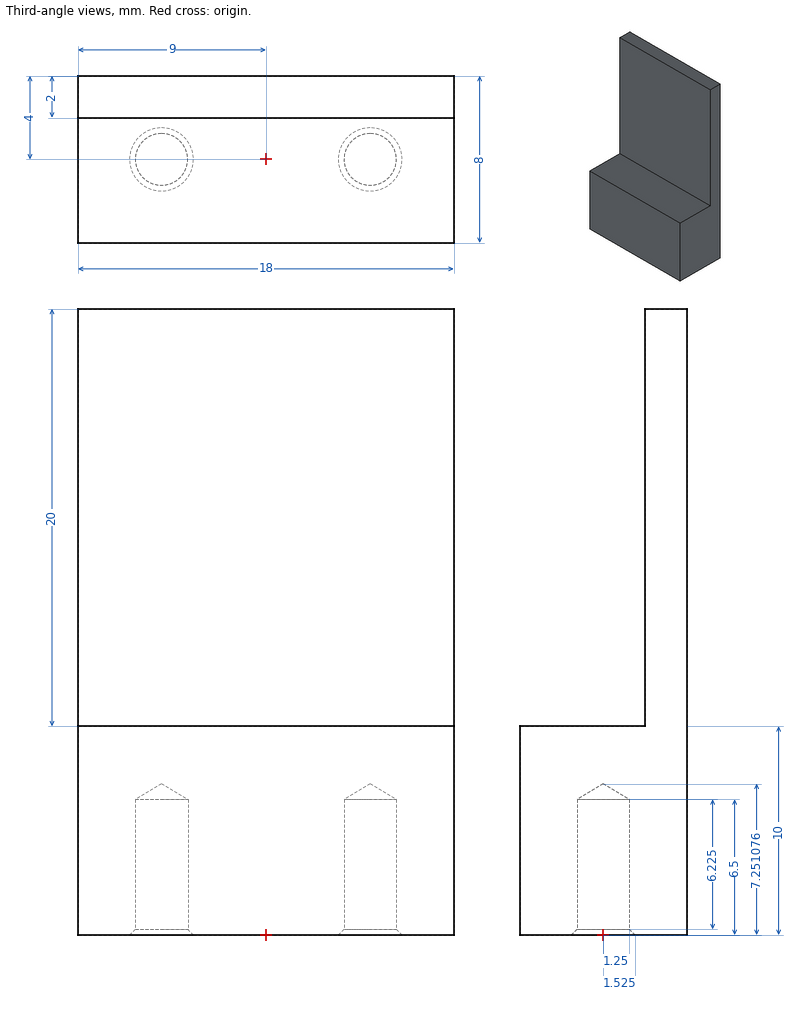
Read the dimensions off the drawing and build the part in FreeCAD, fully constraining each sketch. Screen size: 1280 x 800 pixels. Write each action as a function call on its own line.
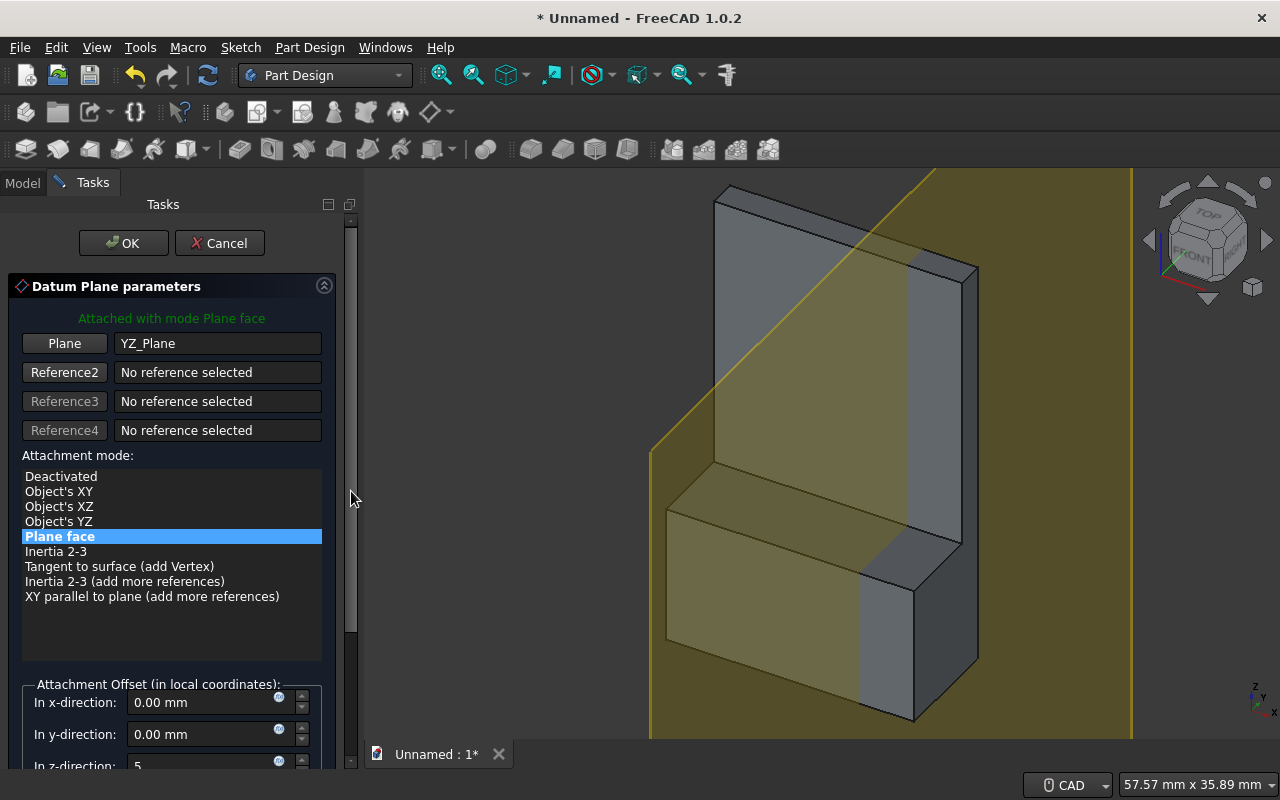
click(124, 243)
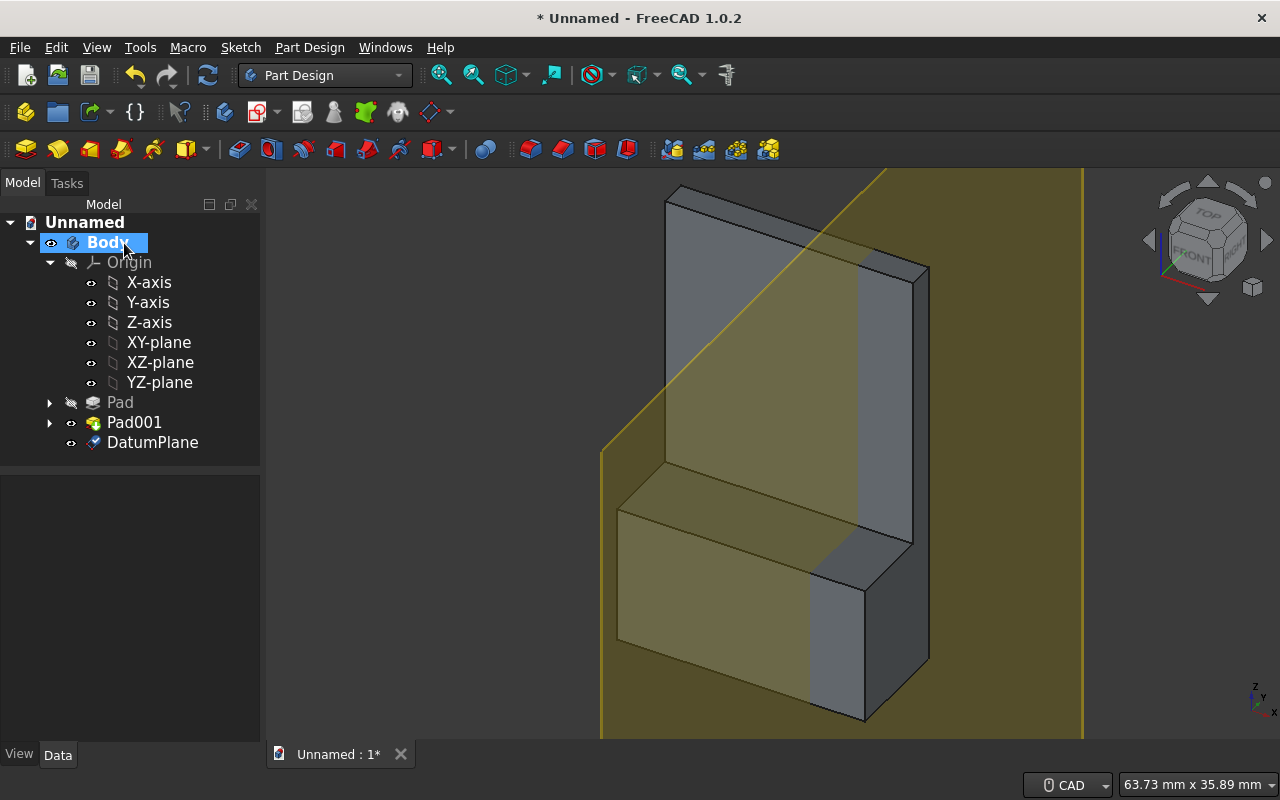
click(116, 443)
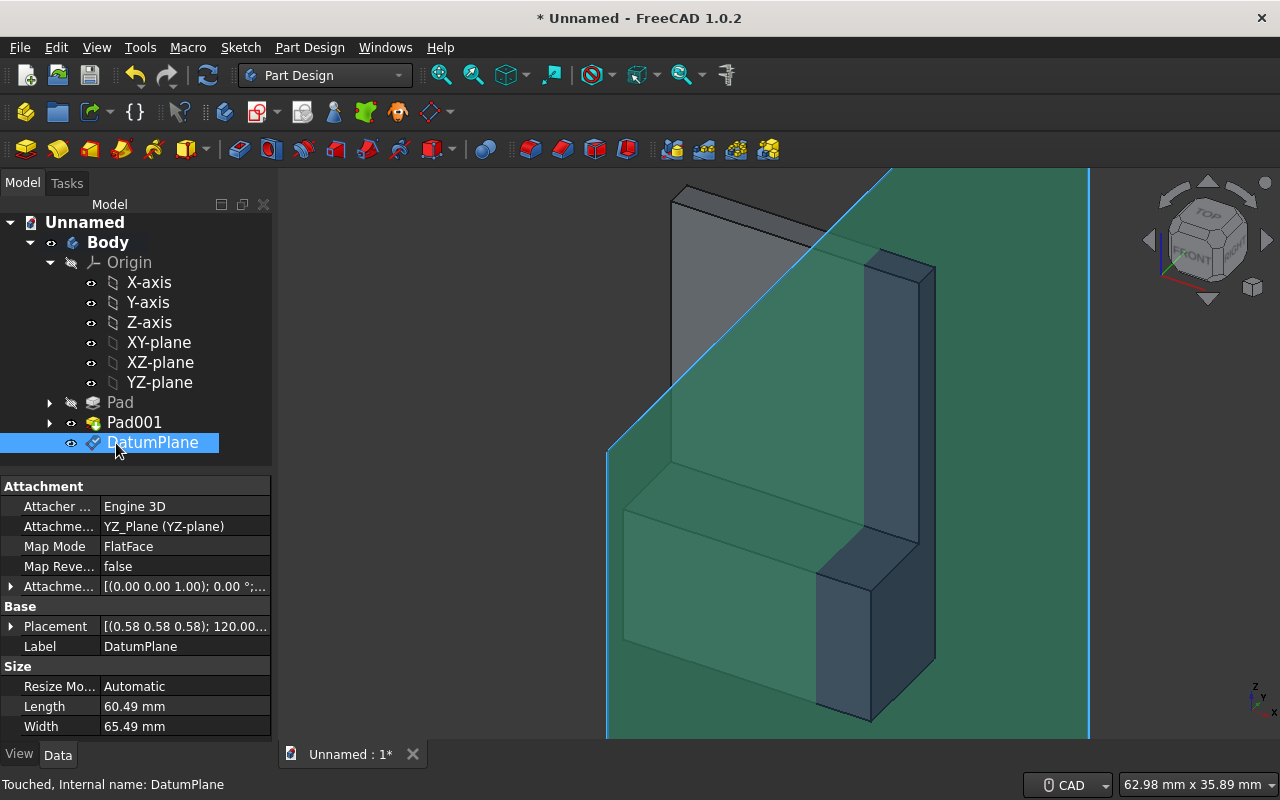
click(258, 112)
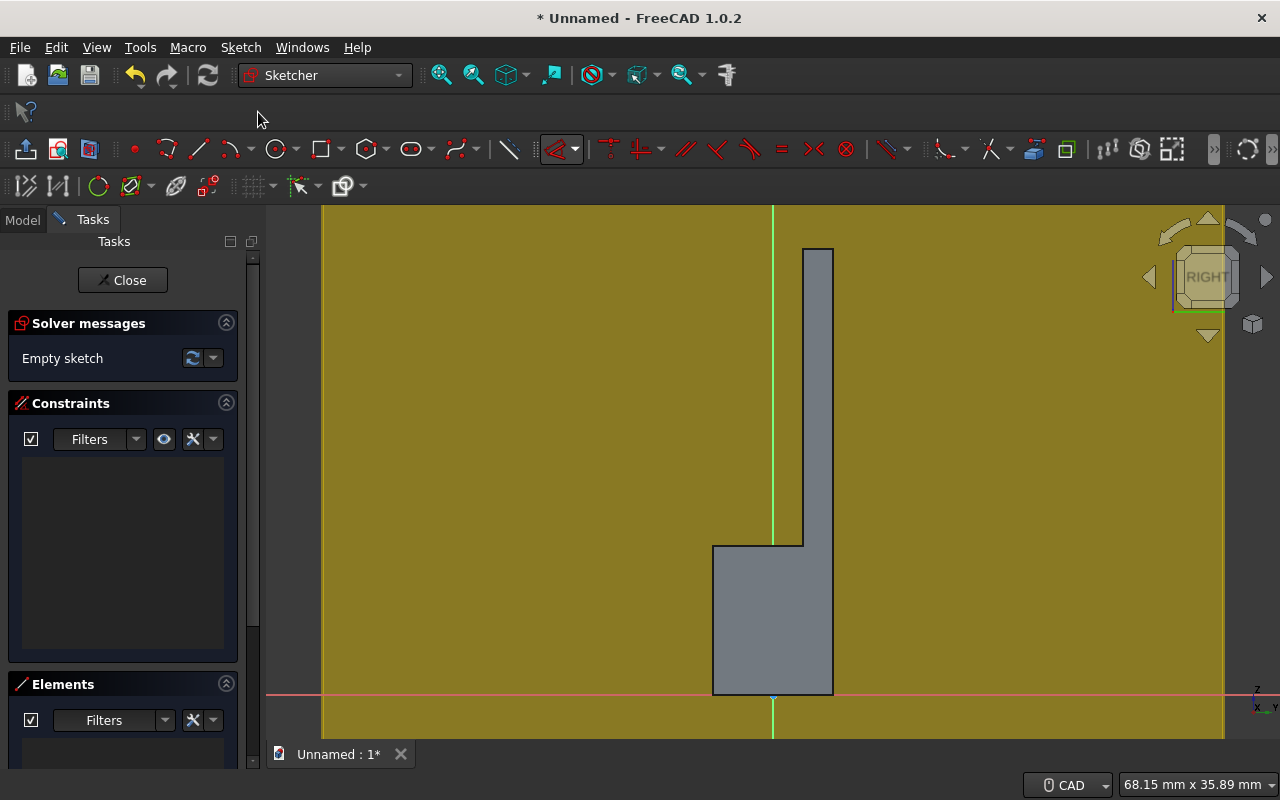
click(90, 150)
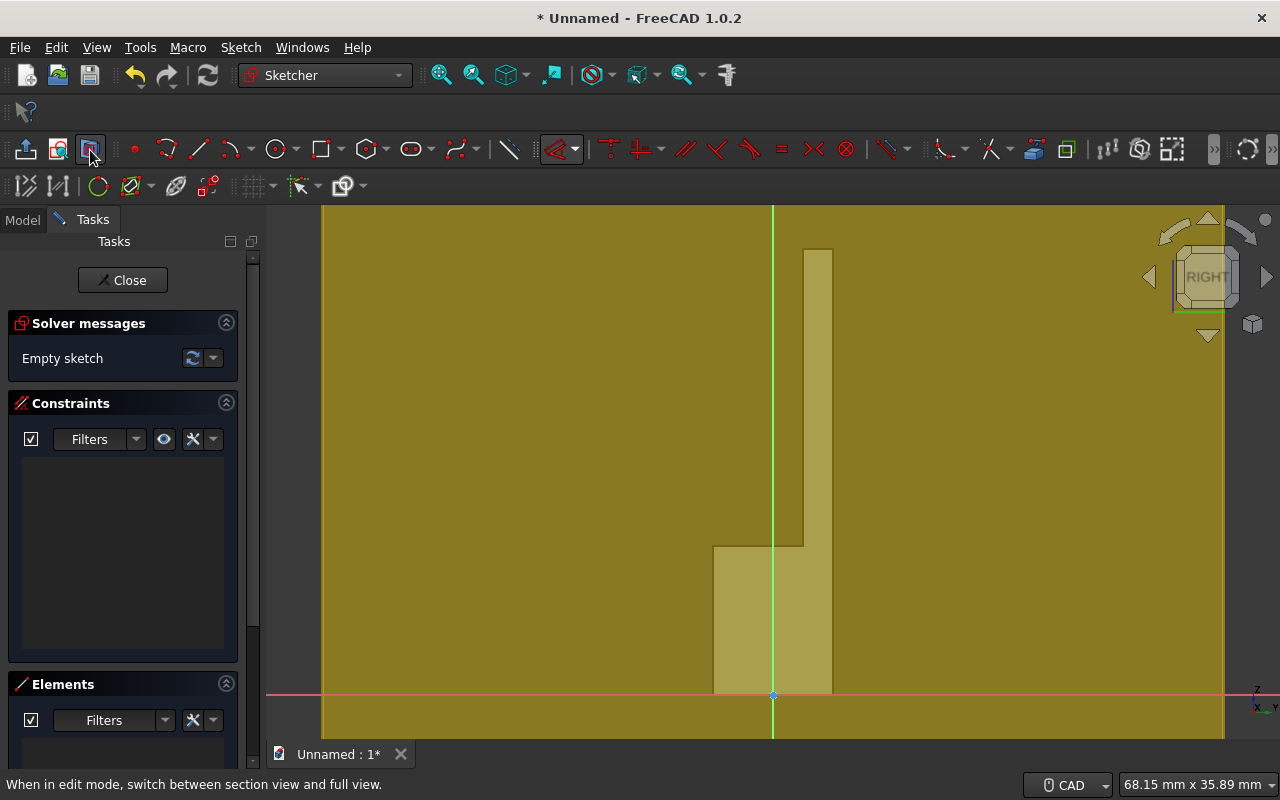
scroll(819, 711, up, 6)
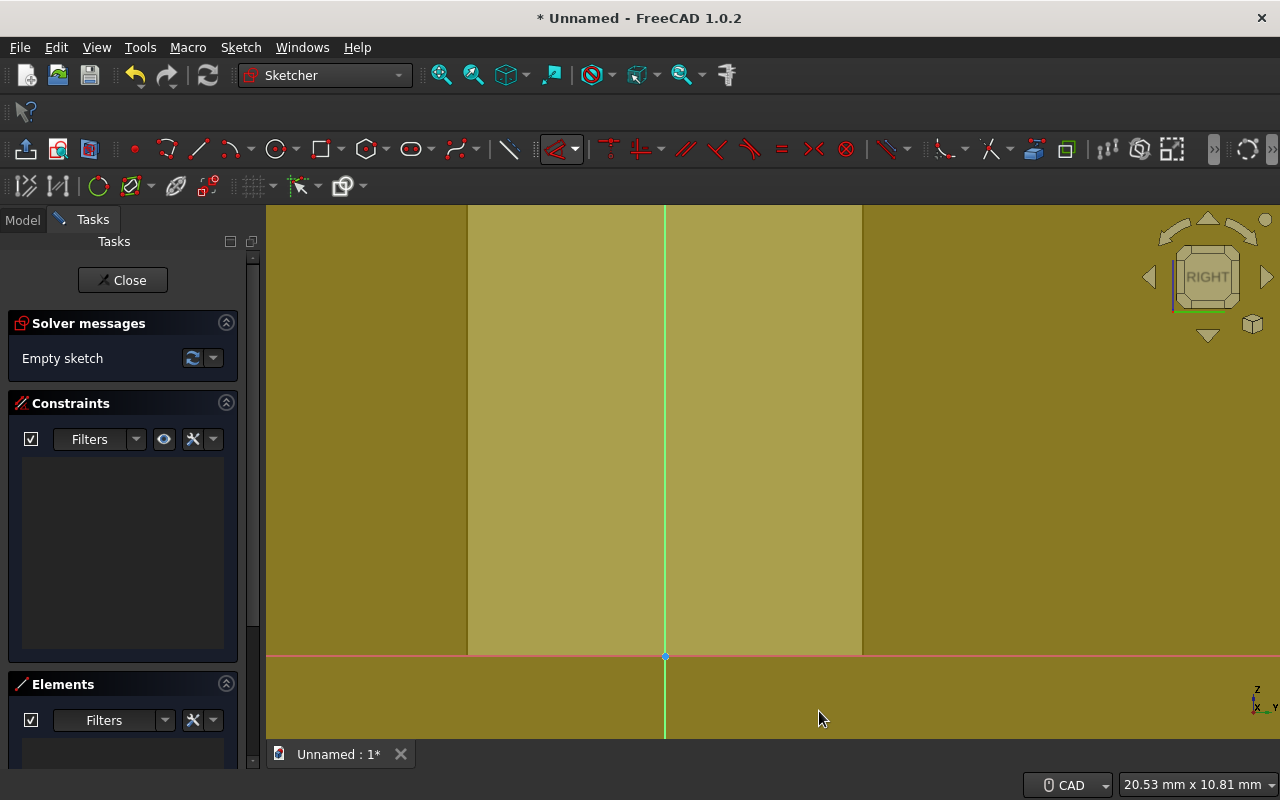
click(168, 150)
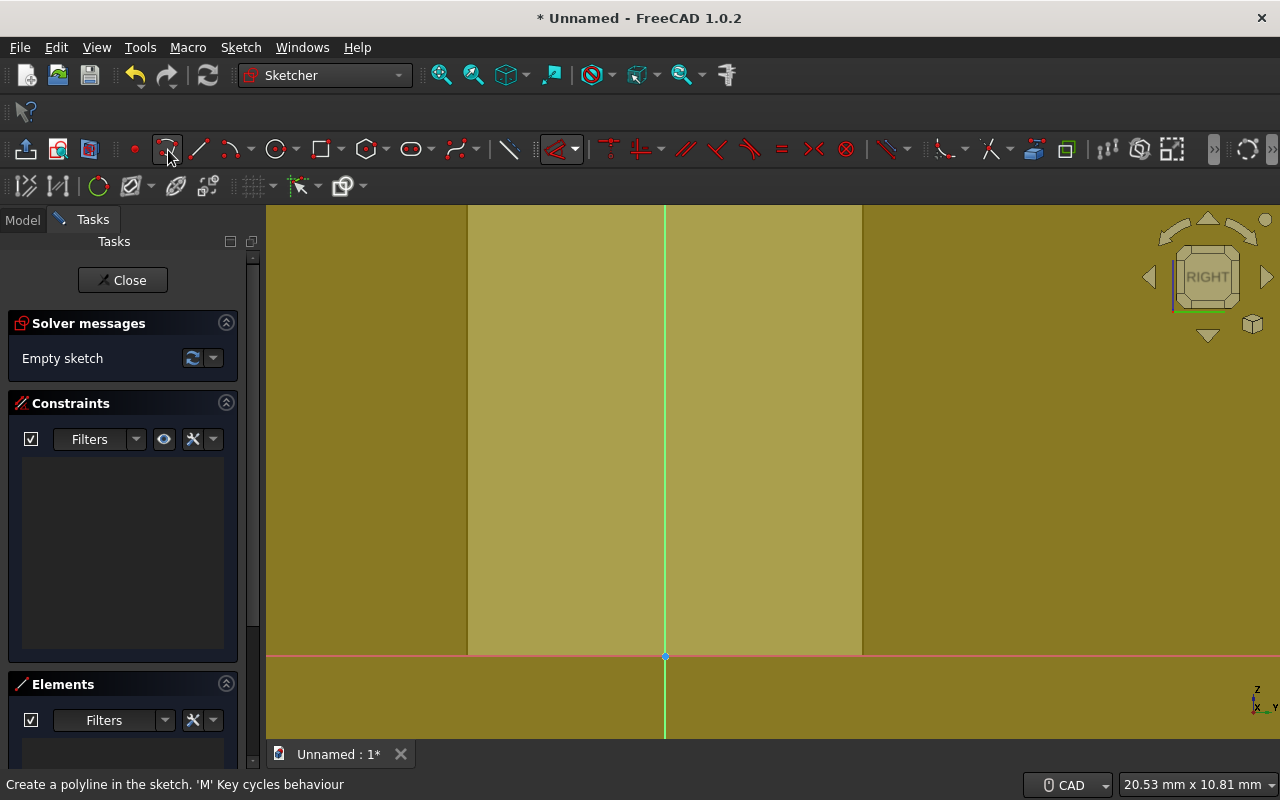
click(665, 656)
click(740, 647)
click(727, 643)
click(727, 335)
click(674, 298)
click(665, 656)
key(Escape)
key(Escape)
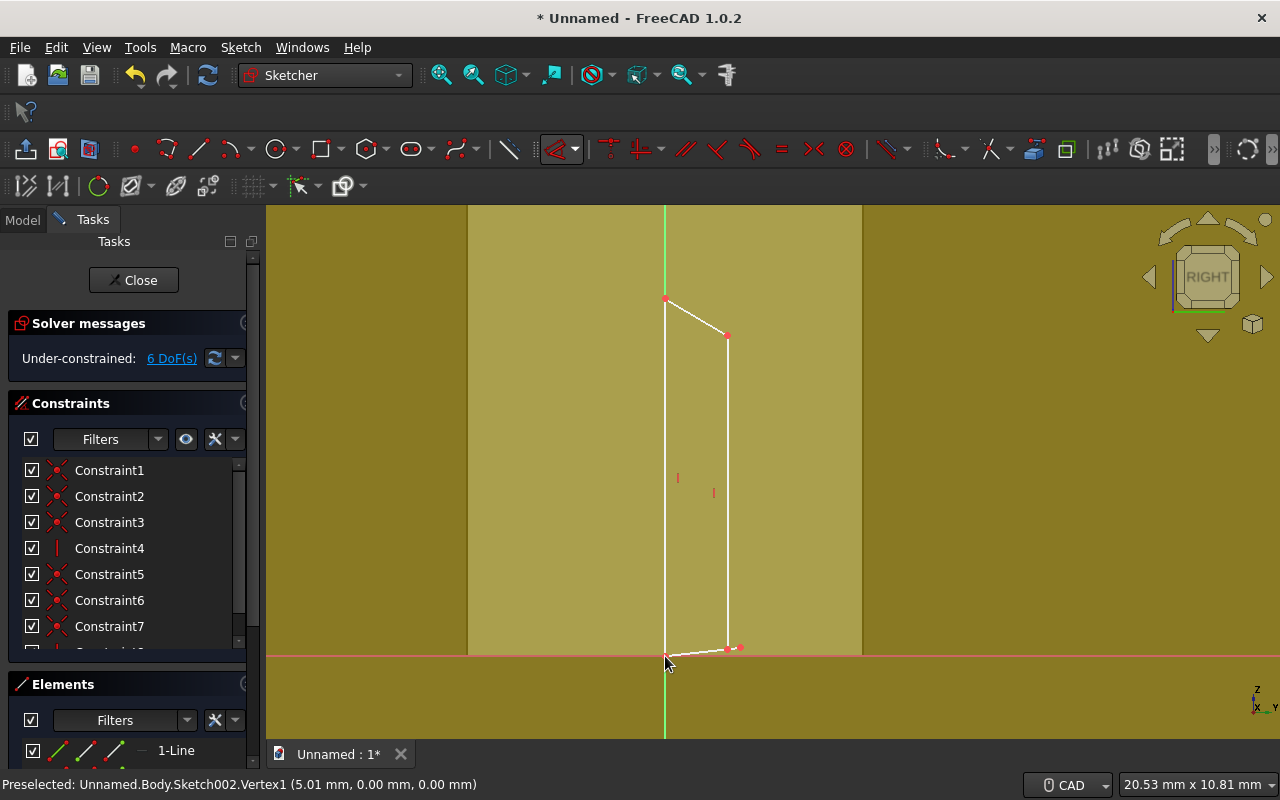
click(688, 654)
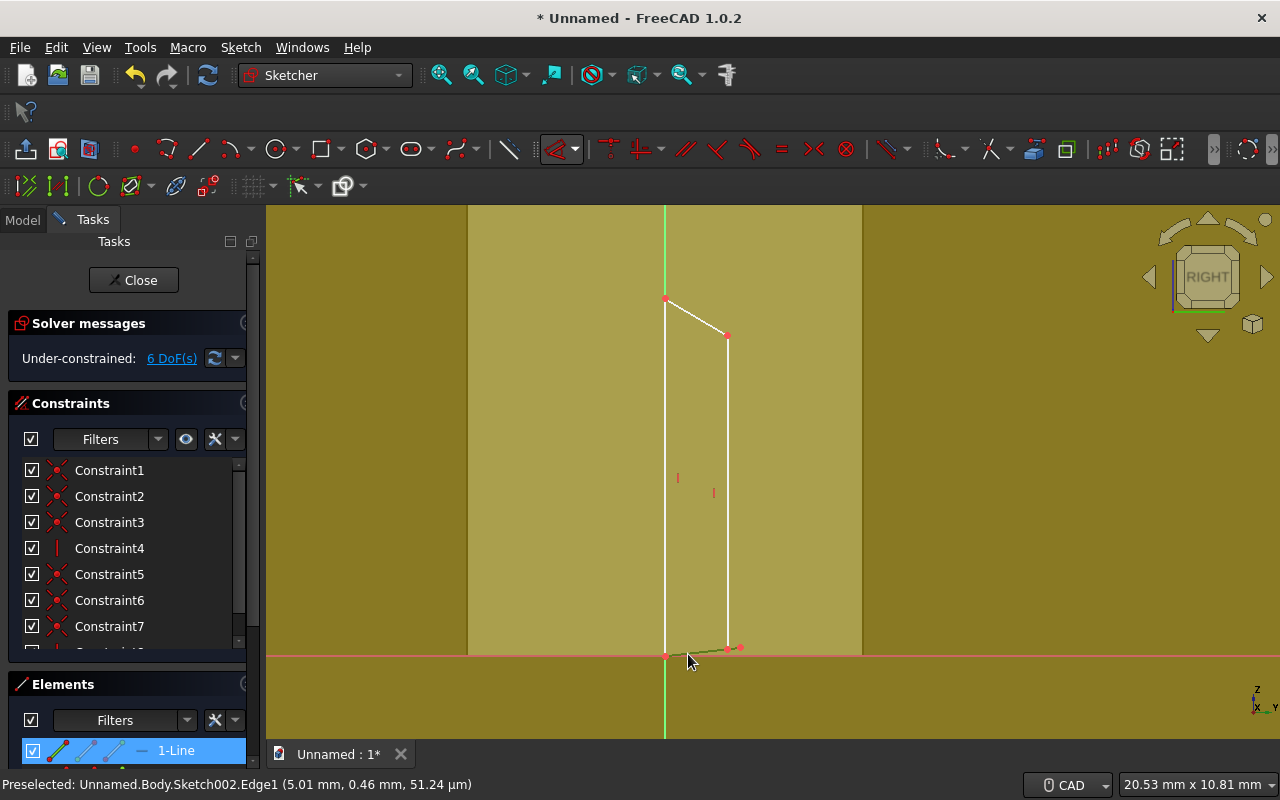
click(664, 150)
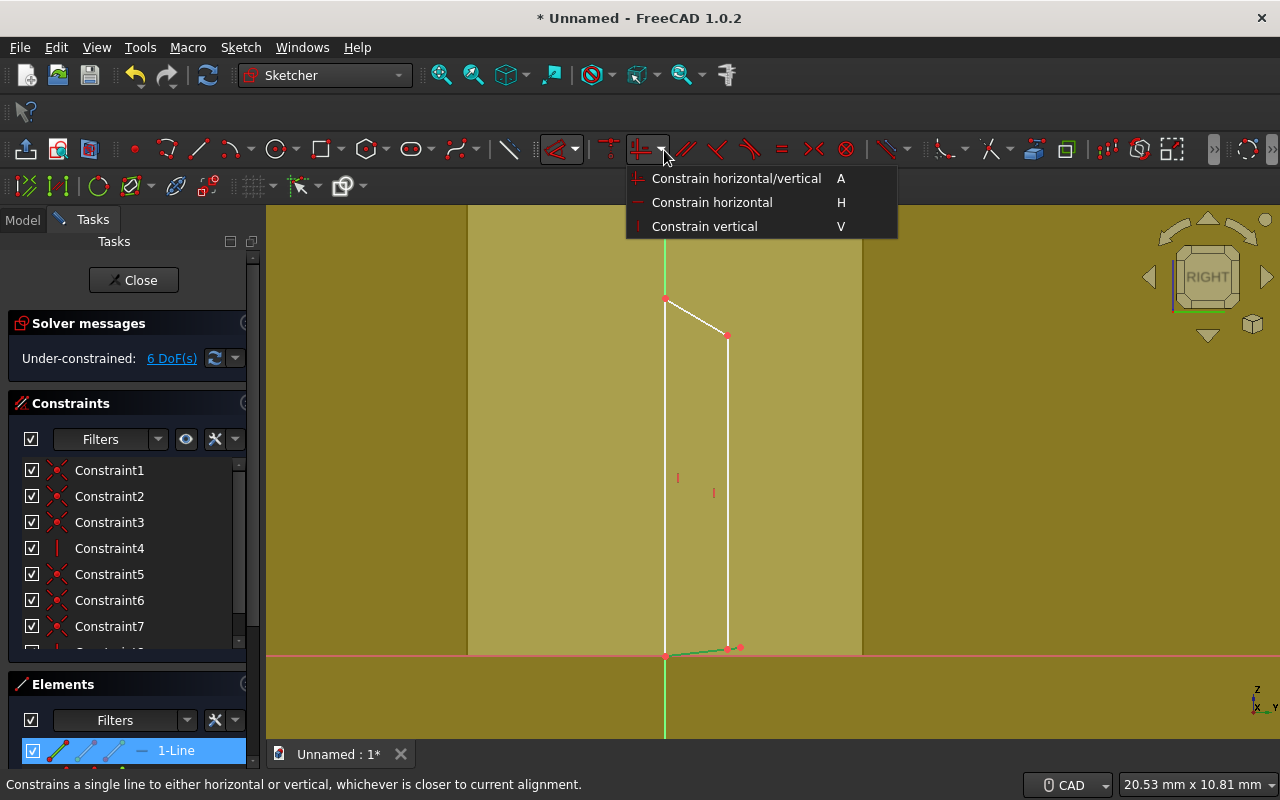
click(762, 202)